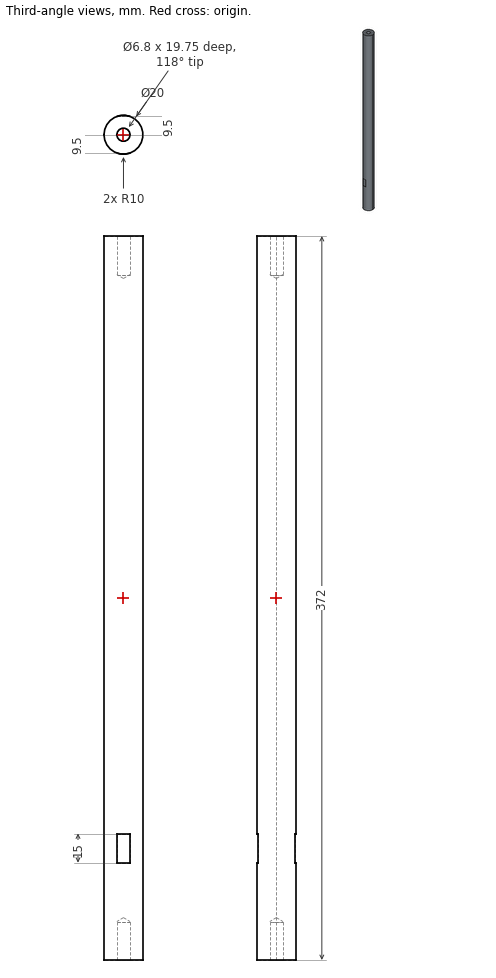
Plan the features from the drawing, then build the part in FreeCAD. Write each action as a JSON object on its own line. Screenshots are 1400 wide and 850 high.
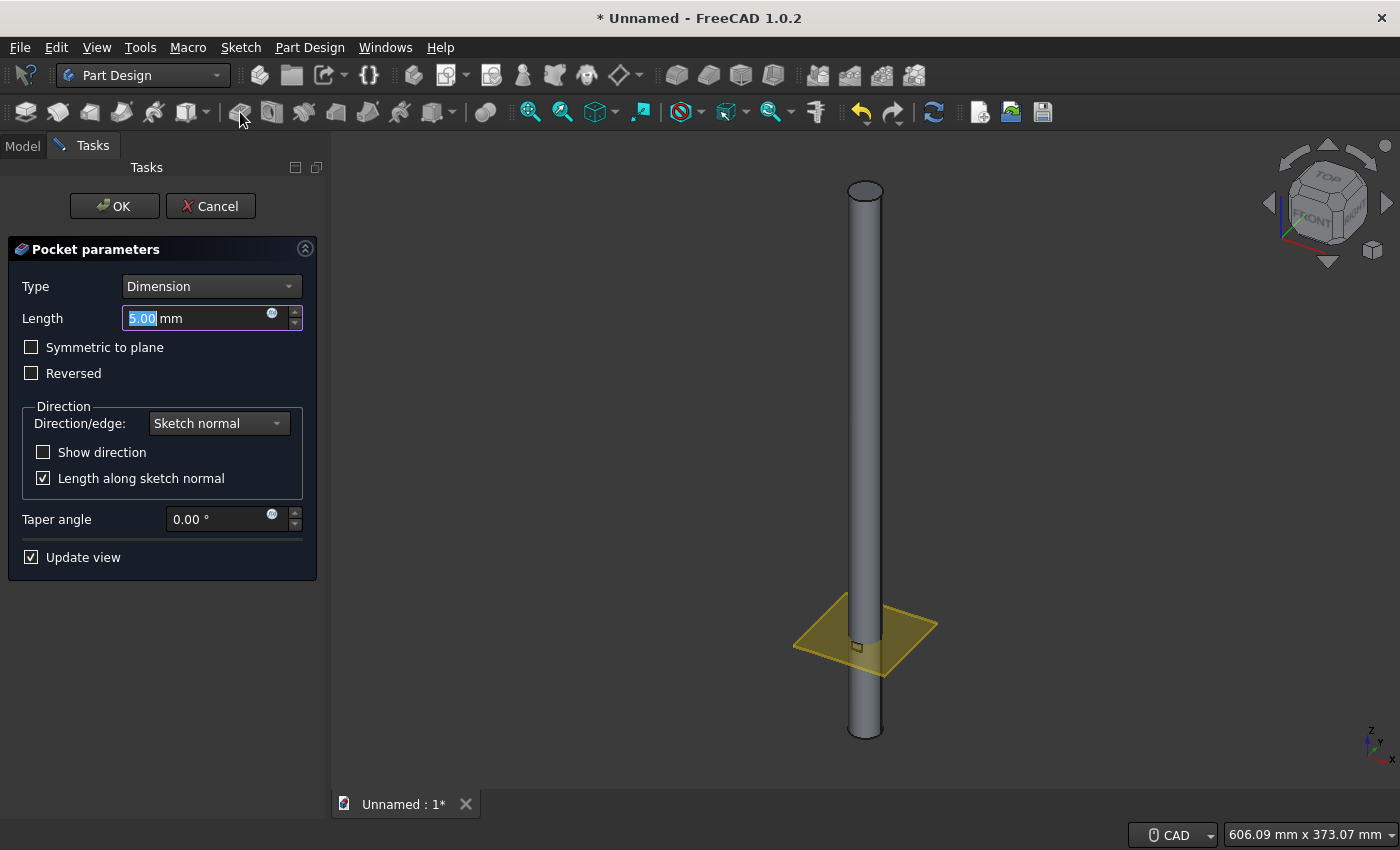
{"action": "type", "text": "15"}
{"action": "key", "text": "Tab"}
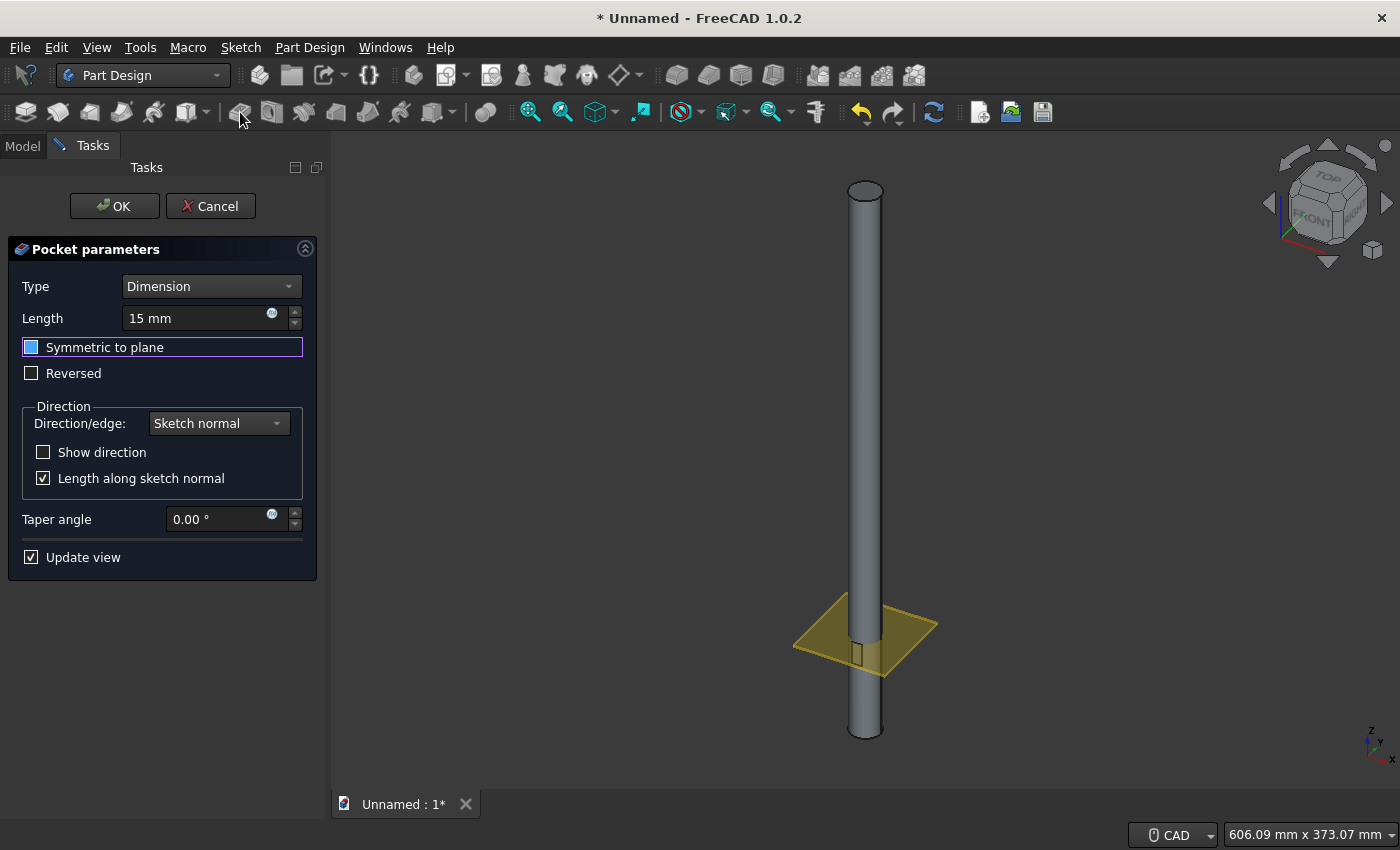
{"action": "left_click", "coordinate": [115, 206]}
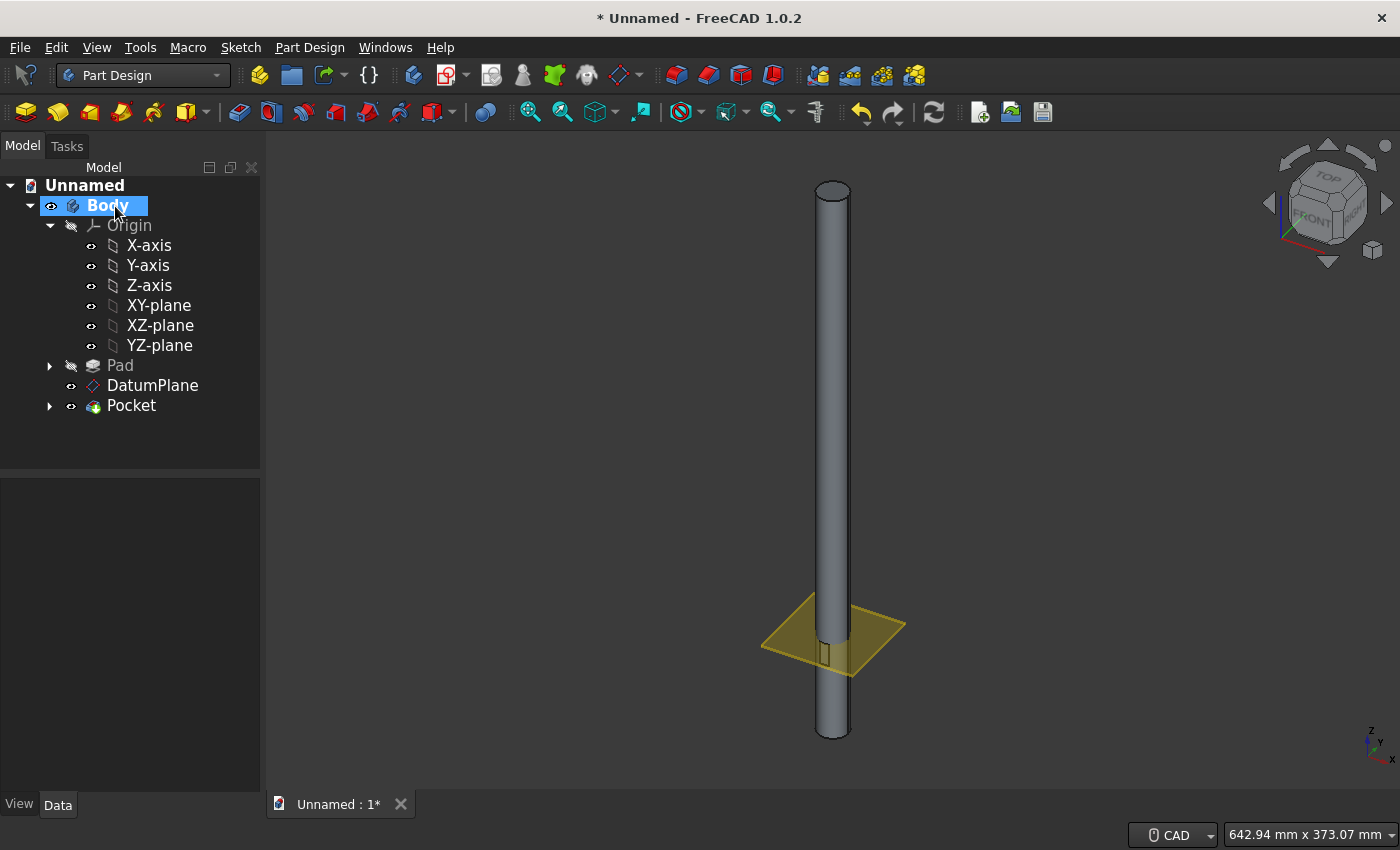
{"action": "left_click", "coordinate": [116, 386]}
{"action": "key", "text": "space"}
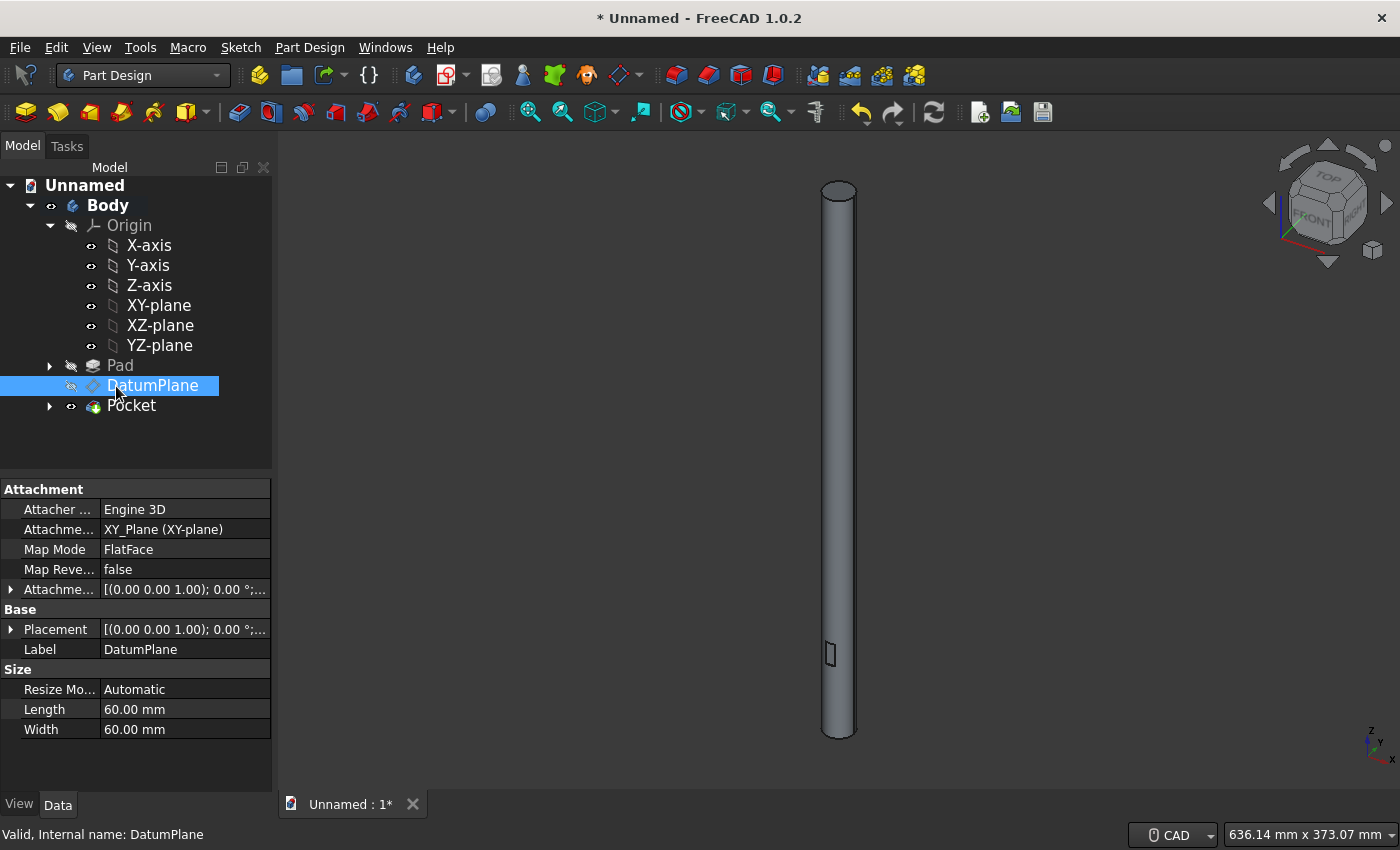
{"action": "key", "text": "5"}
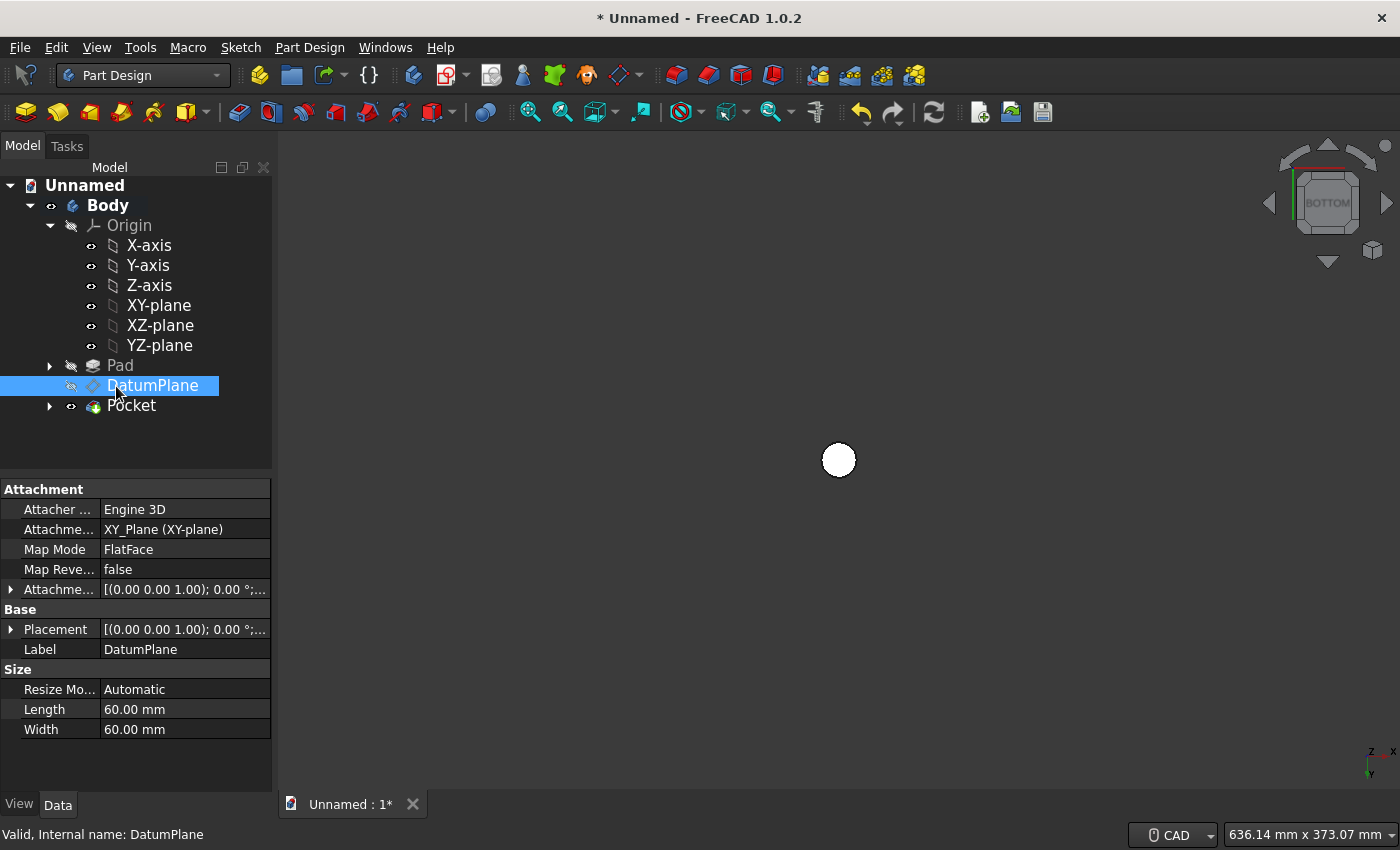
{"action": "left_click", "coordinate": [532, 112]}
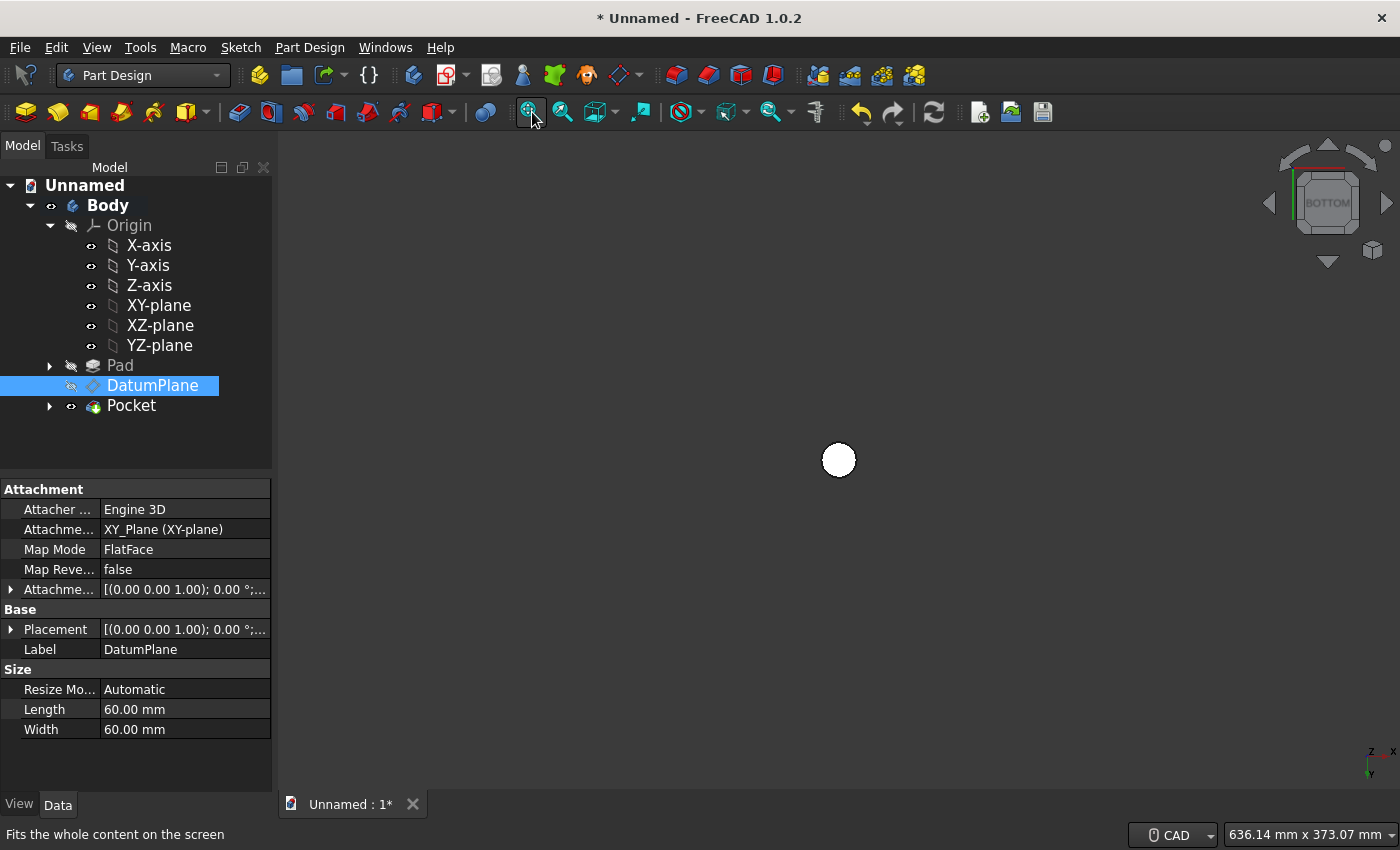
{"action": "left_click", "coordinate": [839, 459]}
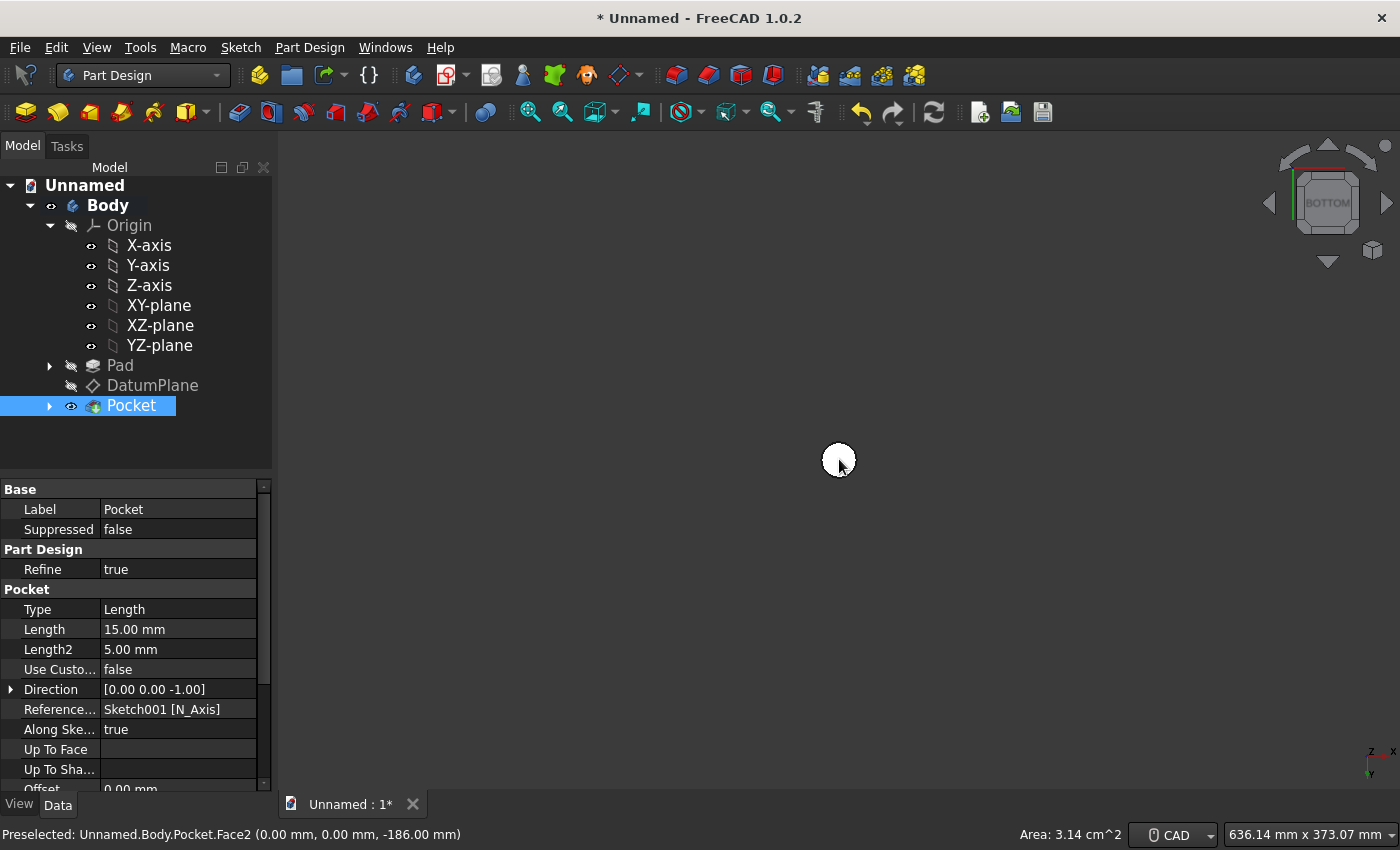
{"action": "left_click", "coordinate": [446, 76]}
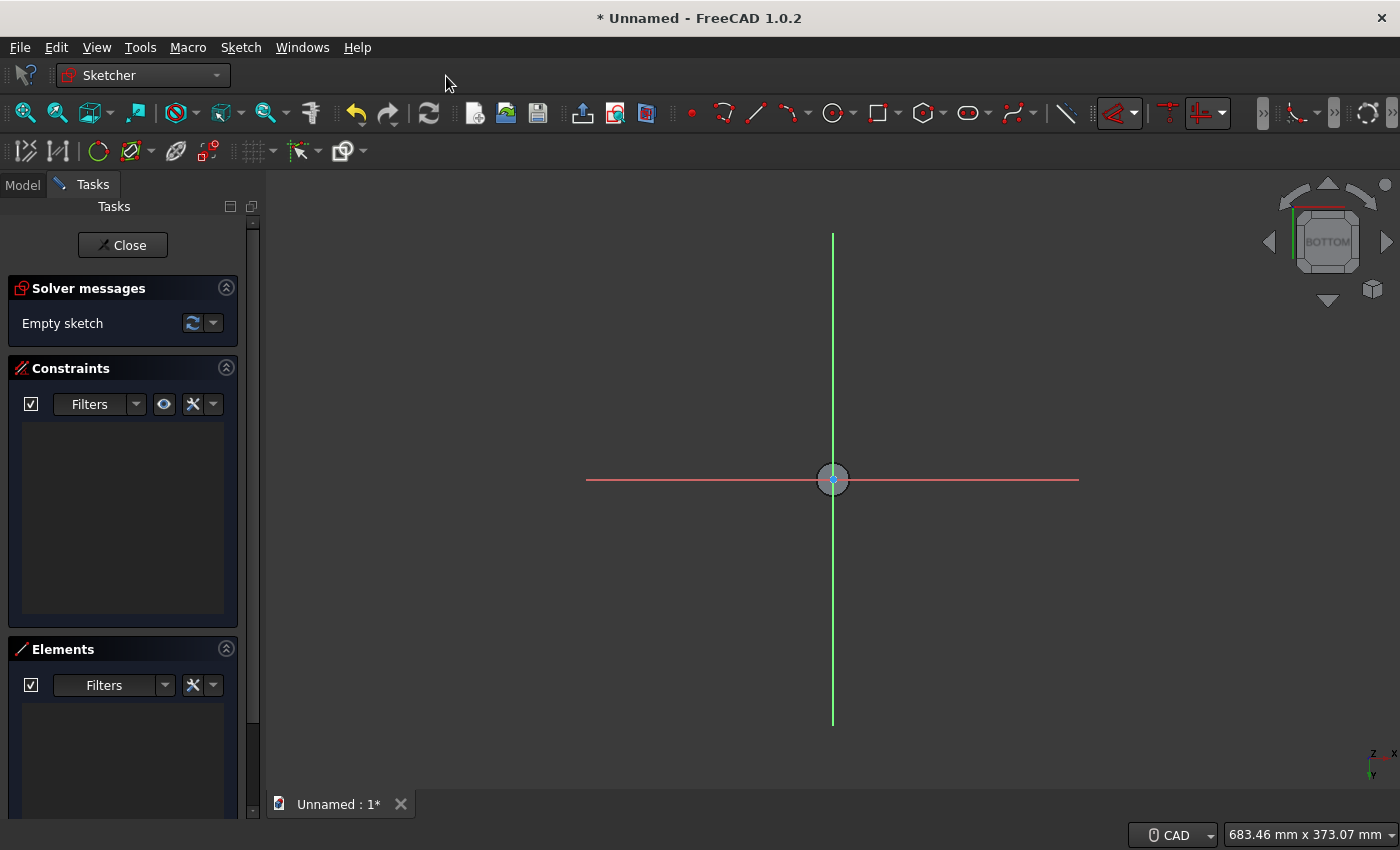
{"action": "scroll", "coordinate": [837, 479], "scroll_direction": "up", "scroll_amount": 15}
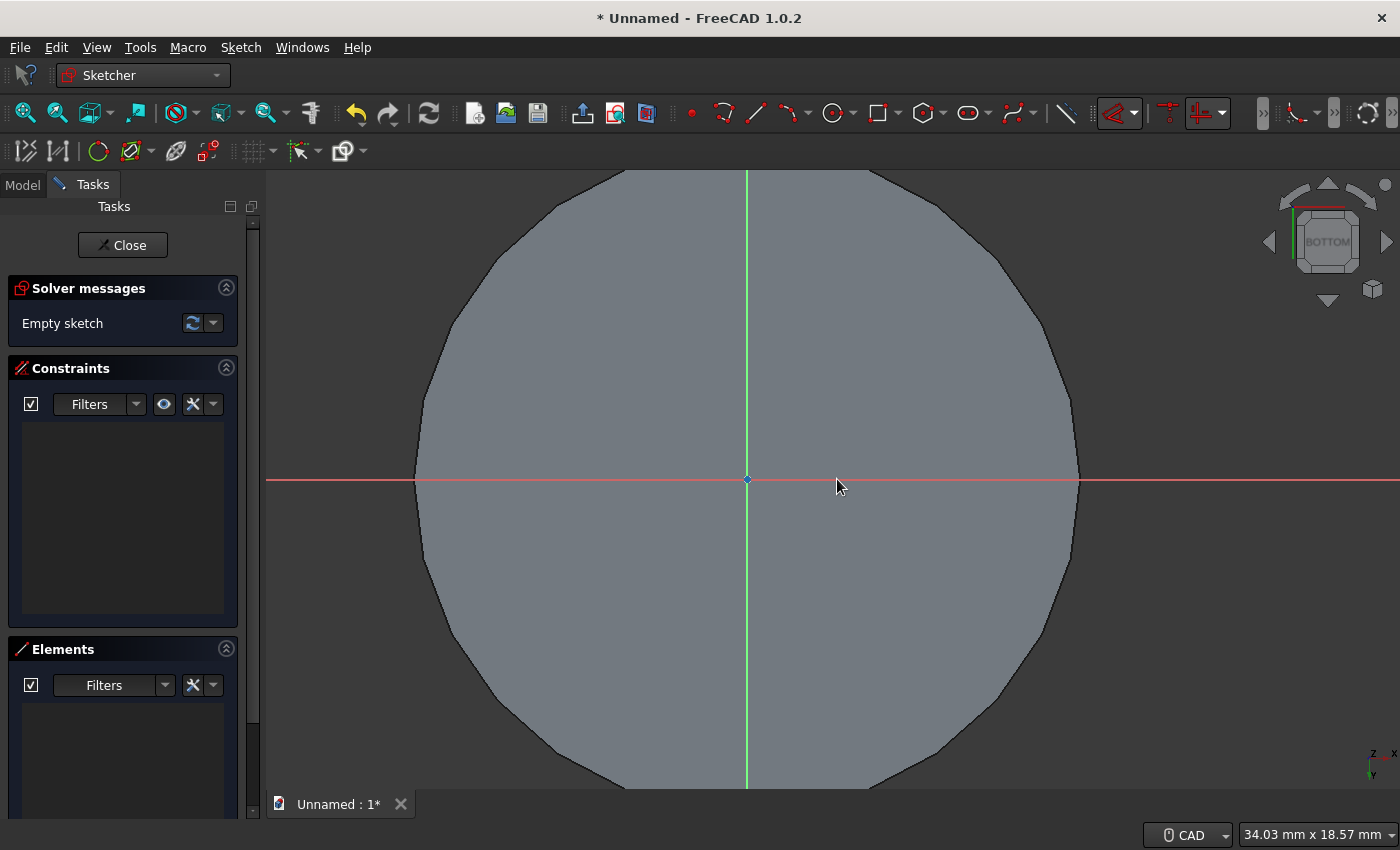
{"action": "scroll", "coordinate": [726, 480], "scroll_direction": "up", "scroll_amount": 3}